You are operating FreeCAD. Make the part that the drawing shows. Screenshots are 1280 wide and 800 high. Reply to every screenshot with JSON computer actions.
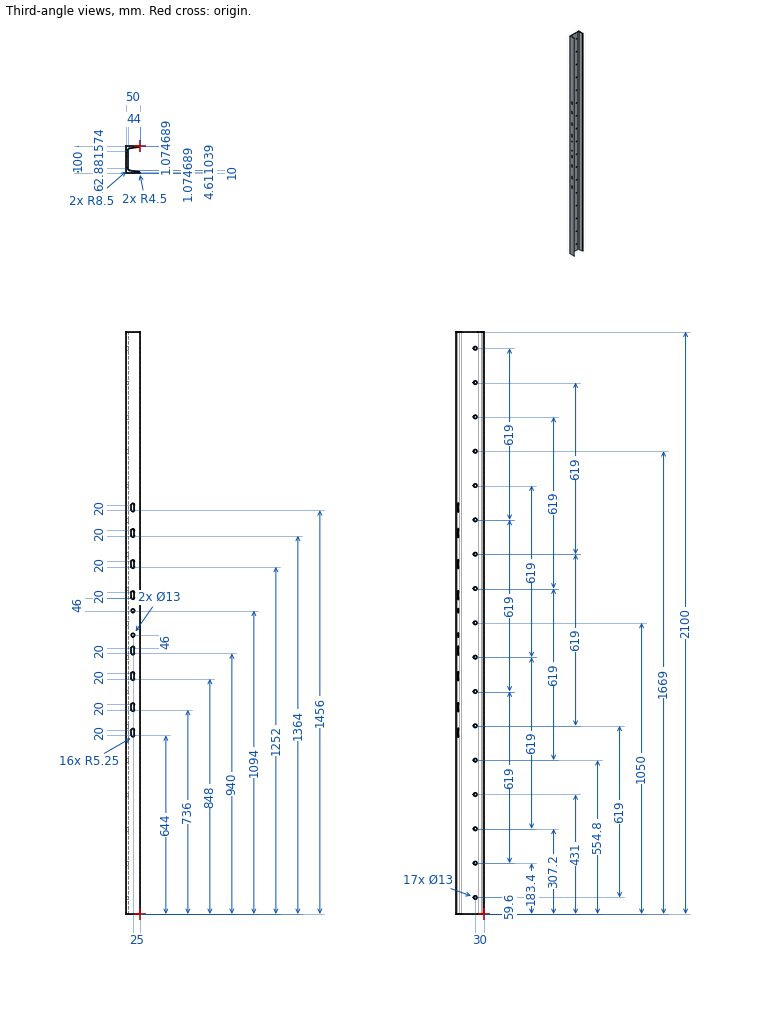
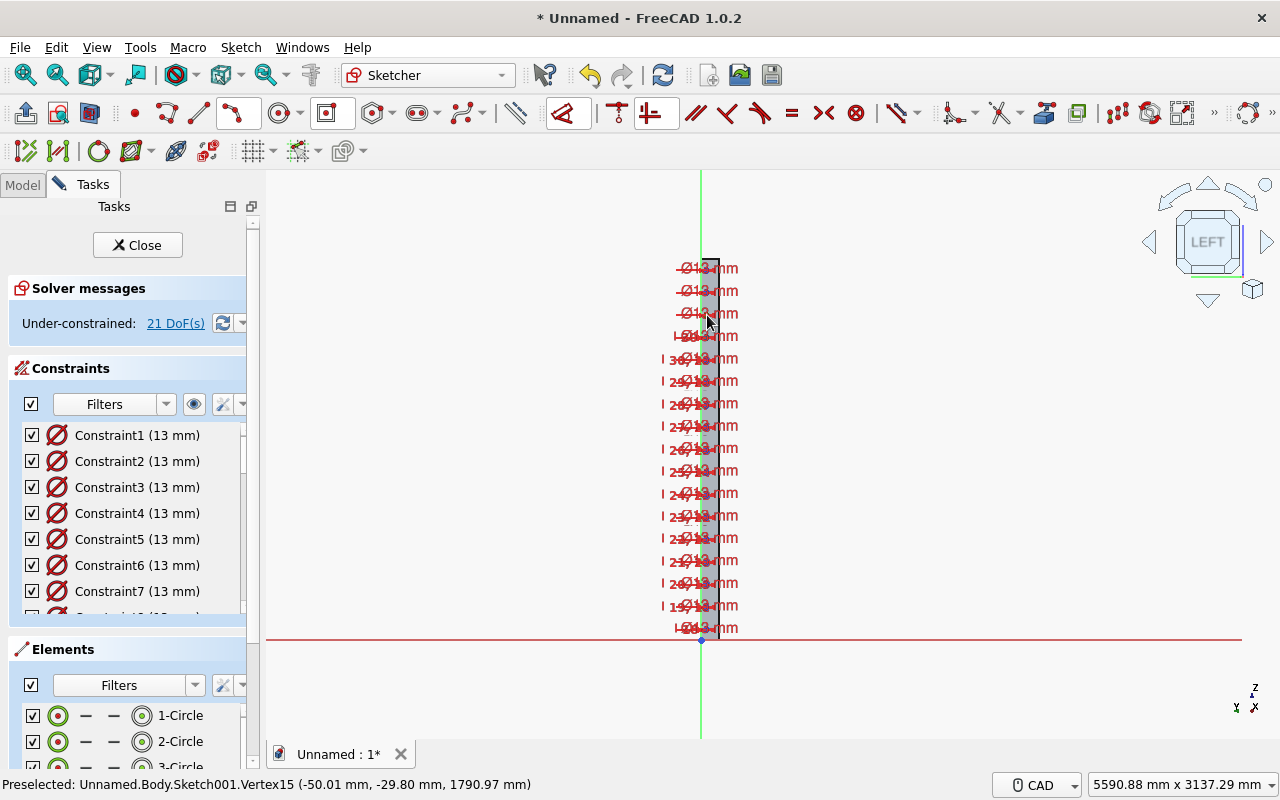
{"action": "key", "text": "v"}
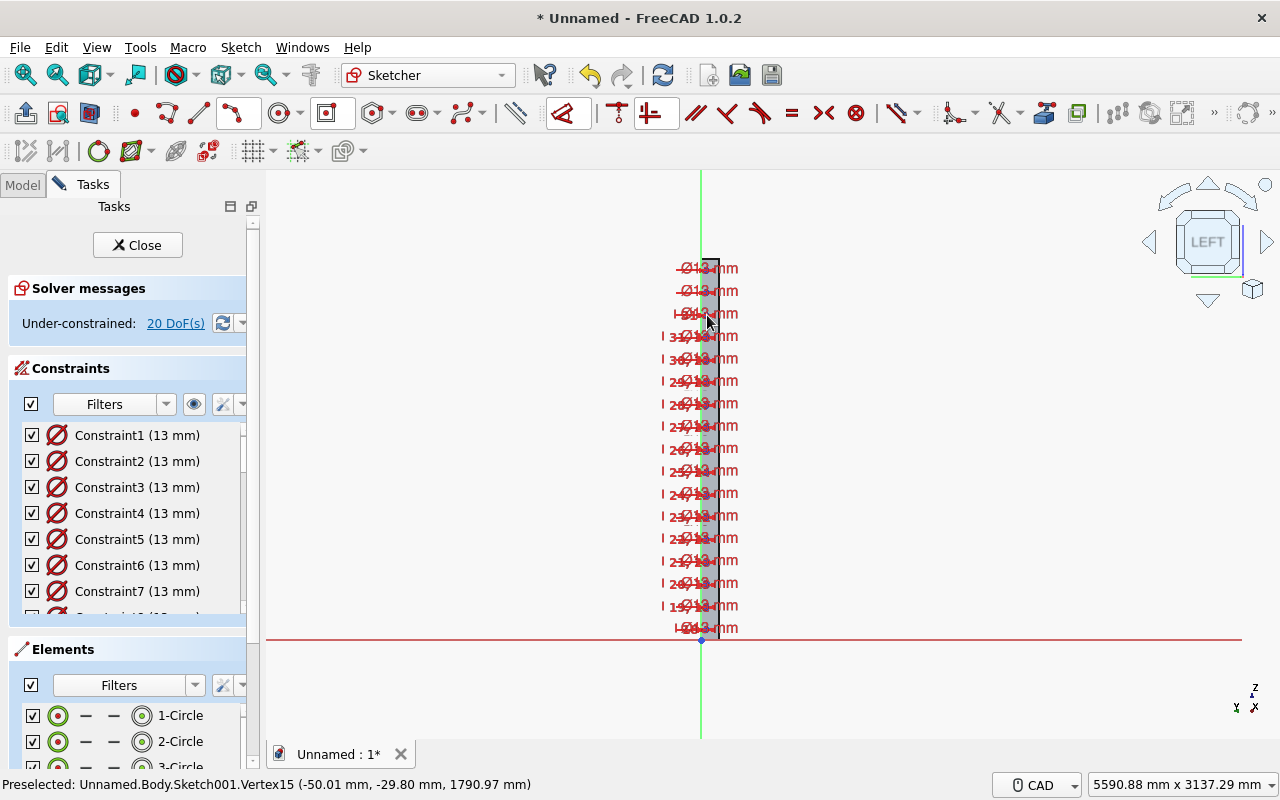
{"action": "left_click", "coordinate": [707, 315]}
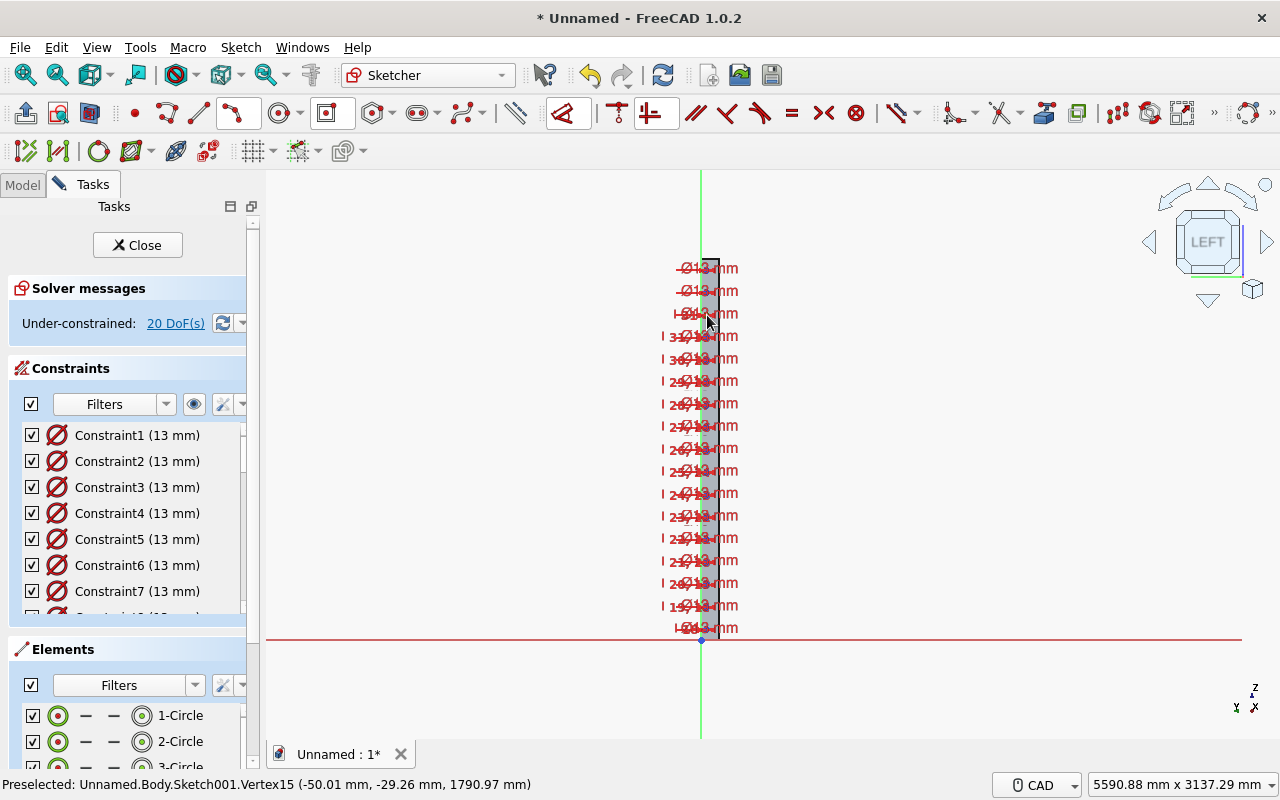
{"action": "left_click", "coordinate": [707, 293]}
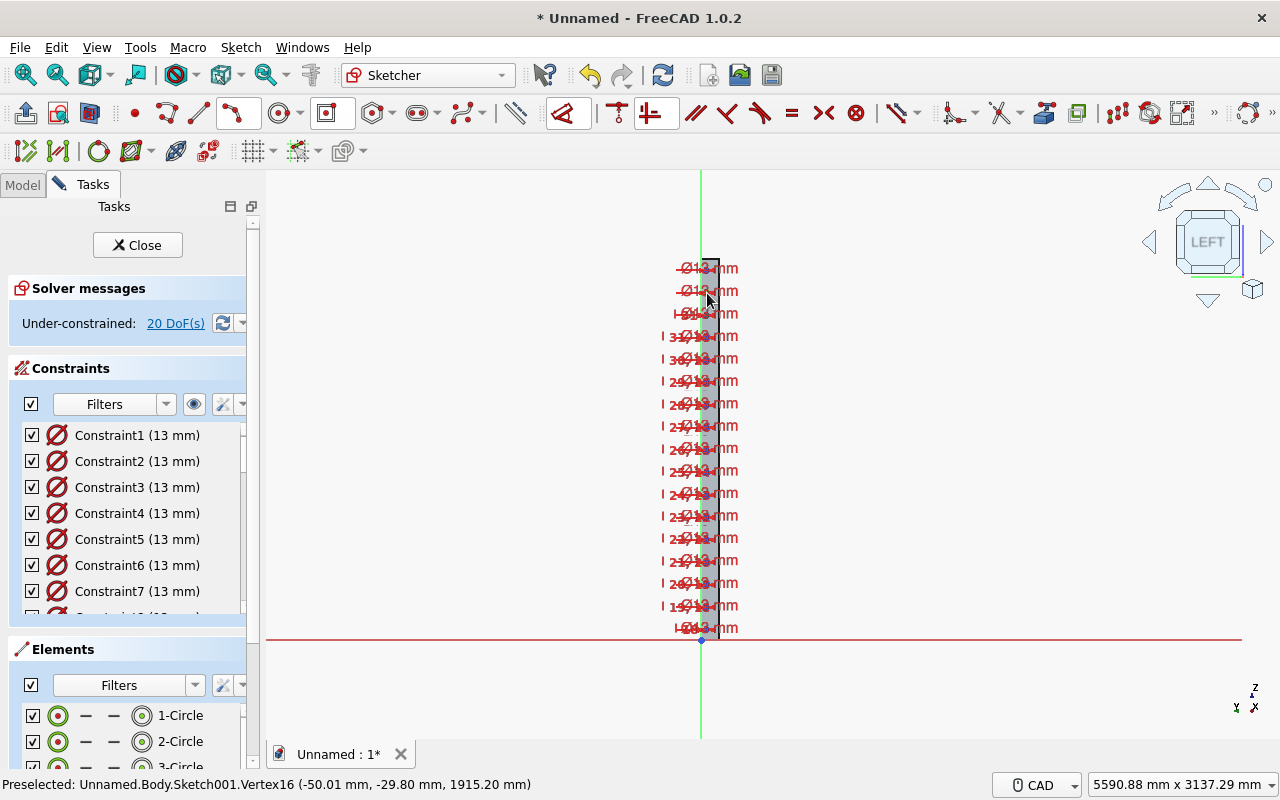
{"action": "key", "text": "v"}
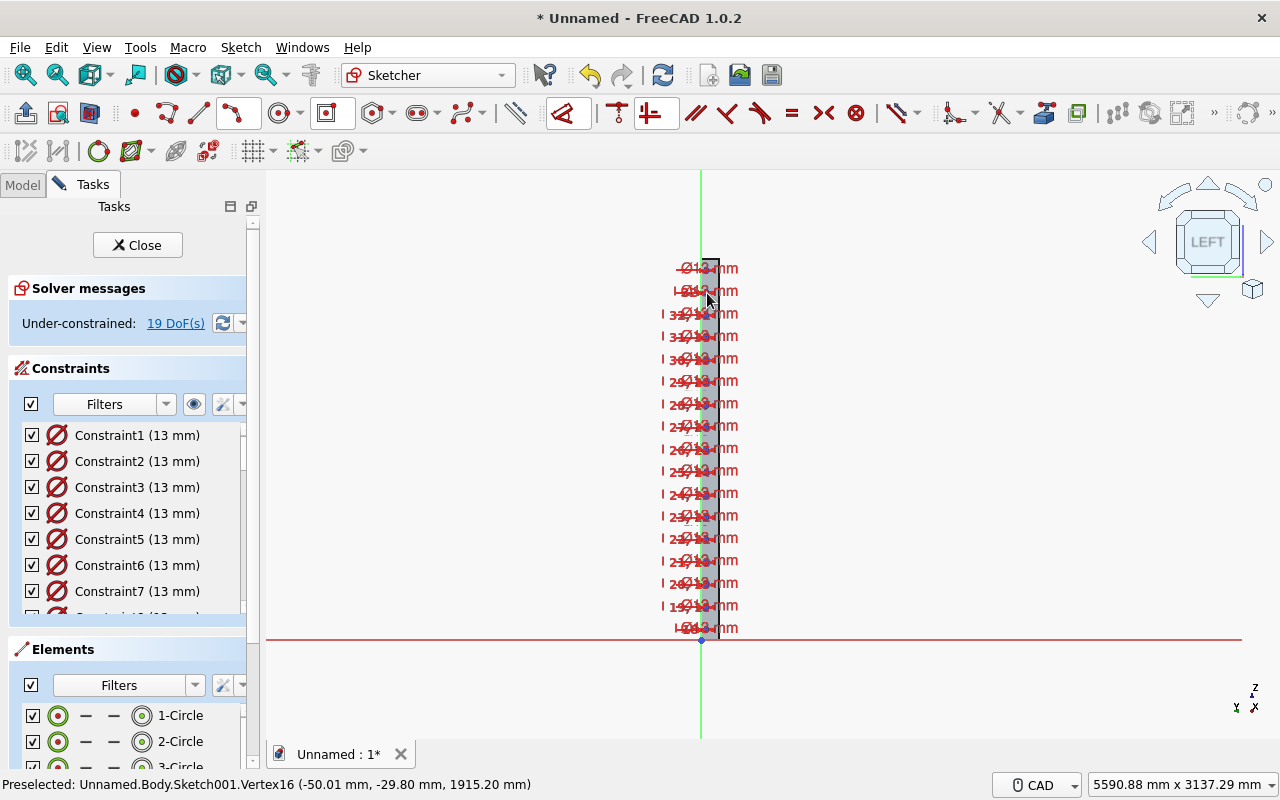
{"action": "left_click", "coordinate": [707, 293]}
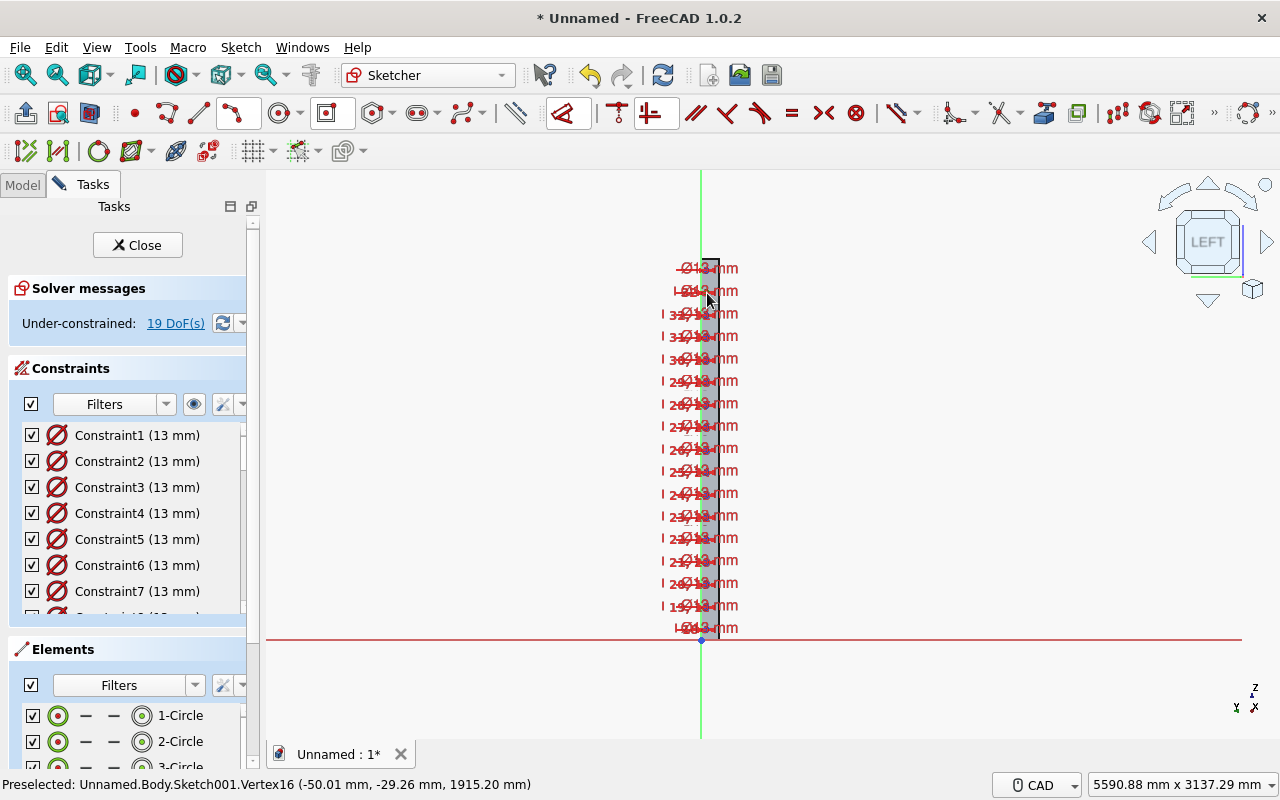
{"action": "left_click", "coordinate": [707, 270]}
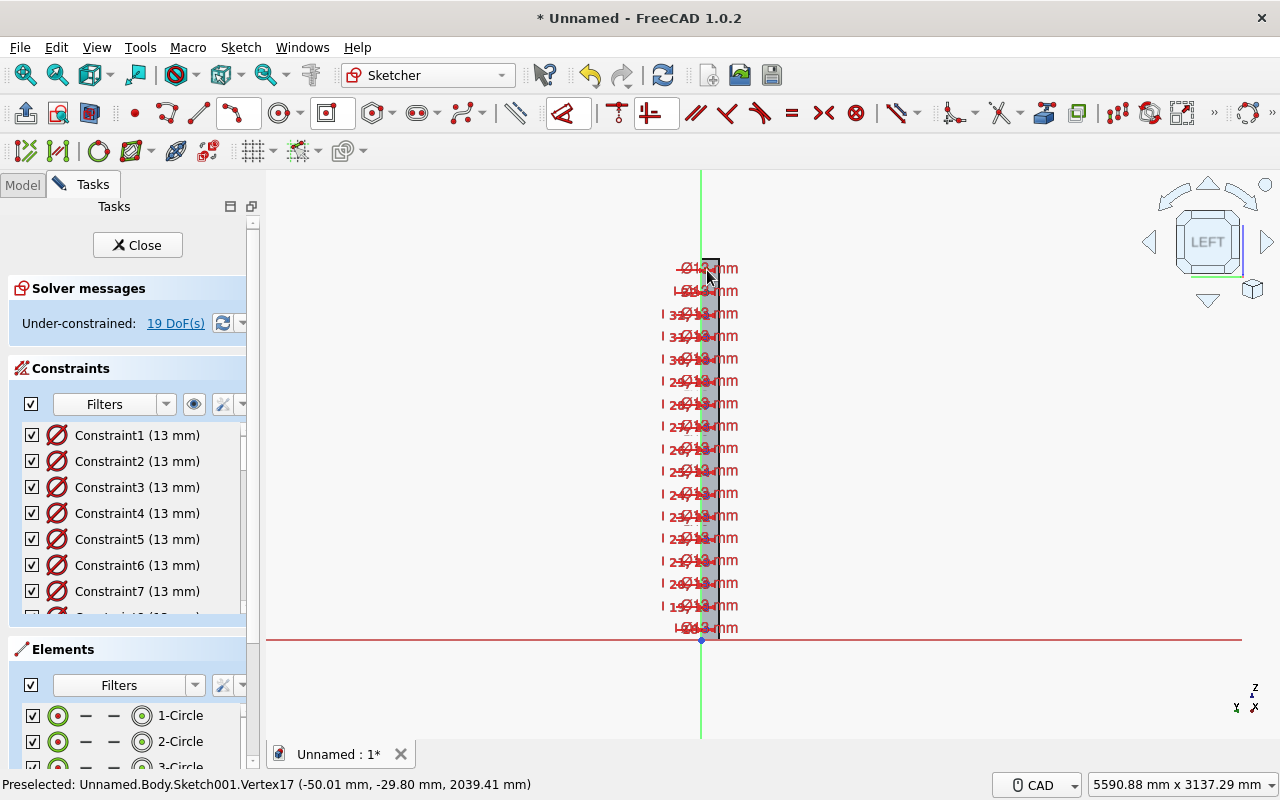
{"action": "key", "text": "v"}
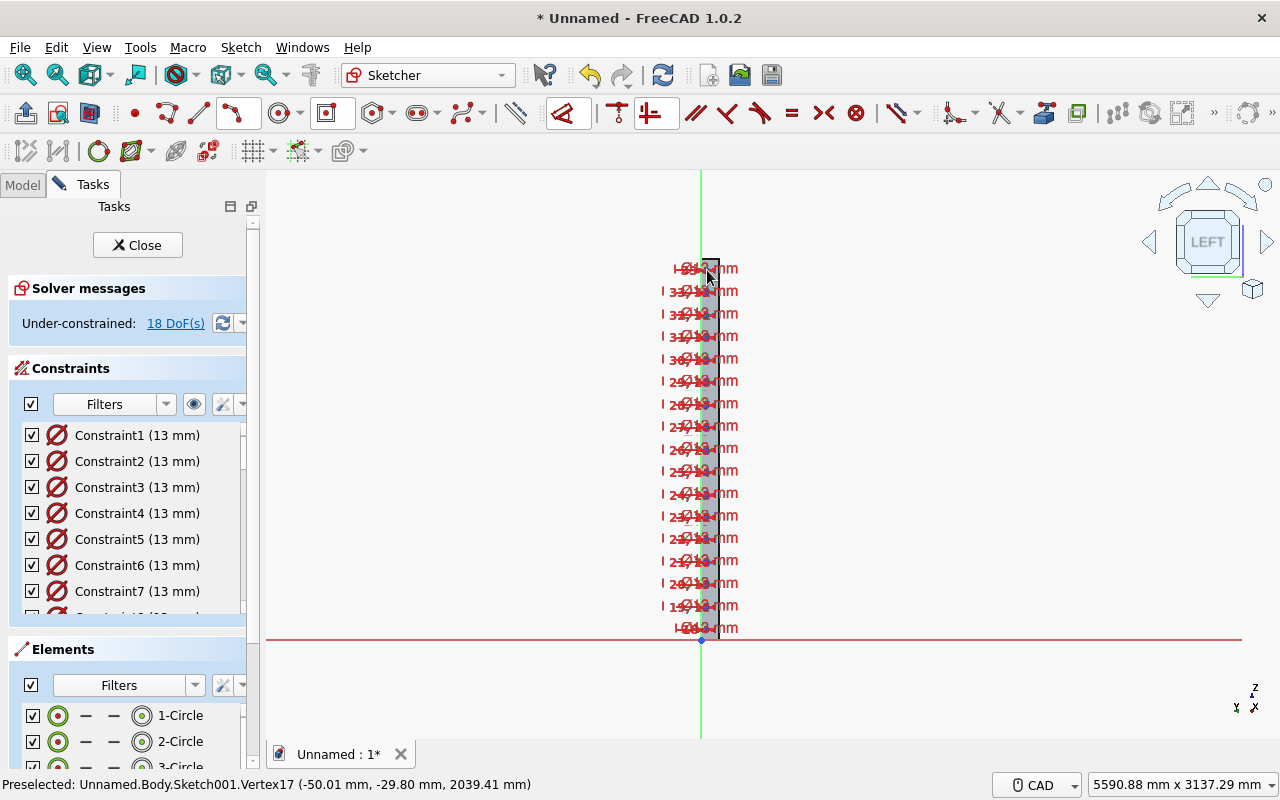
{"action": "left_click", "coordinate": [562, 114]}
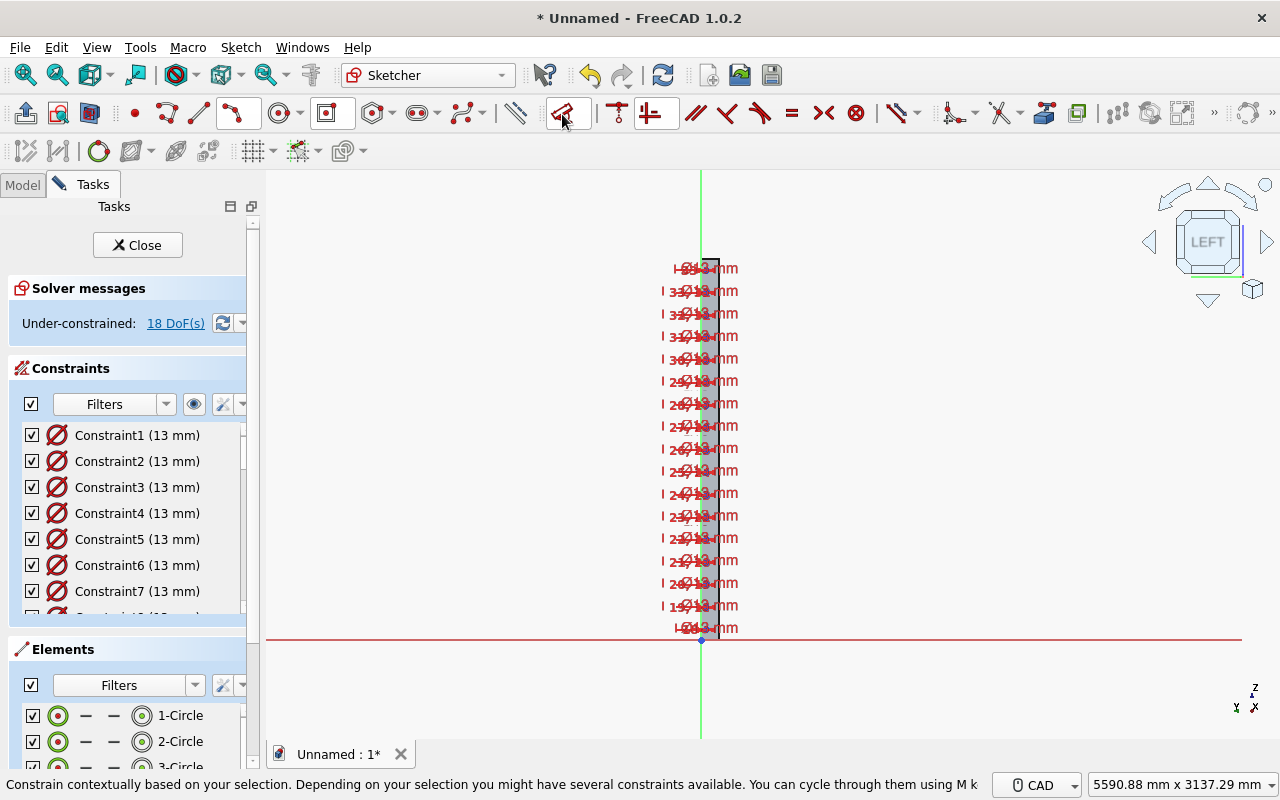
{"action": "scroll", "coordinate": [707, 630], "scroll_direction": "up", "scroll_amount": 10}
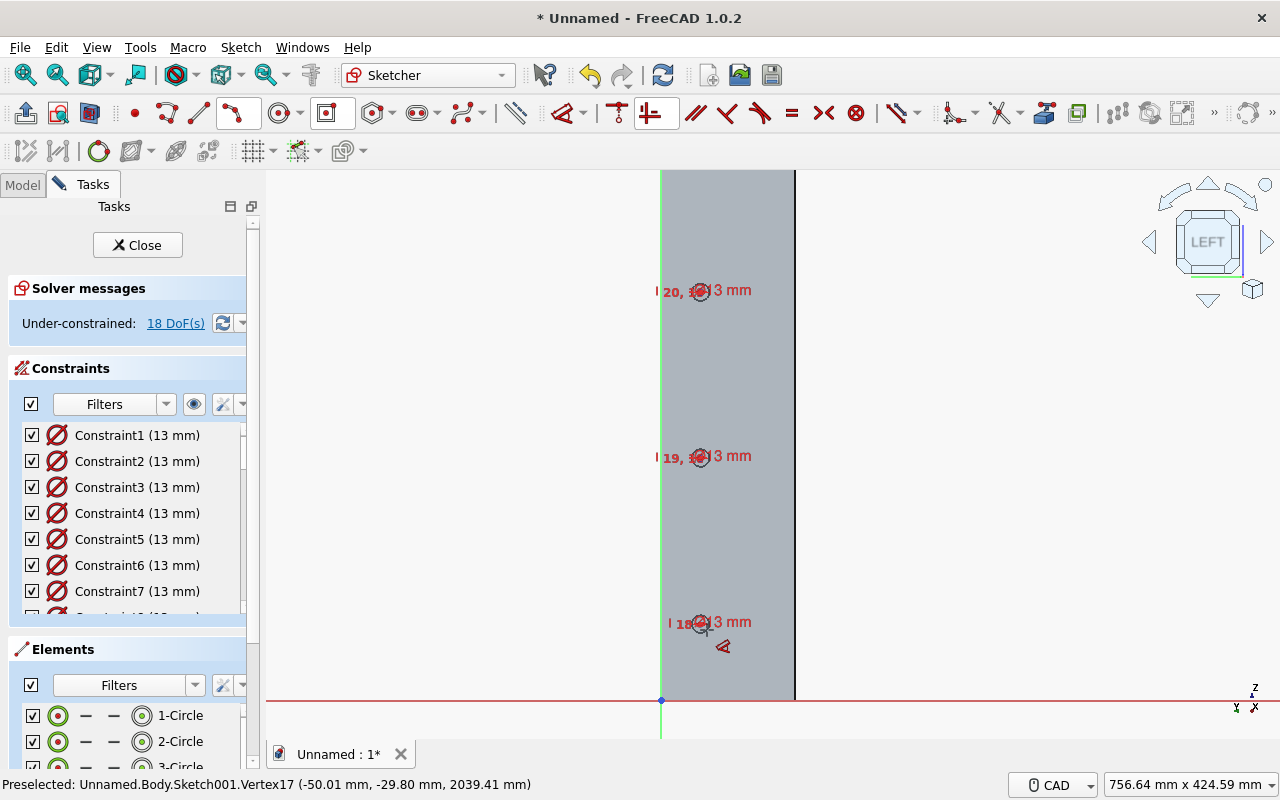
{"action": "left_click", "coordinate": [701, 624]}
{"action": "left_click", "coordinate": [681, 590]}